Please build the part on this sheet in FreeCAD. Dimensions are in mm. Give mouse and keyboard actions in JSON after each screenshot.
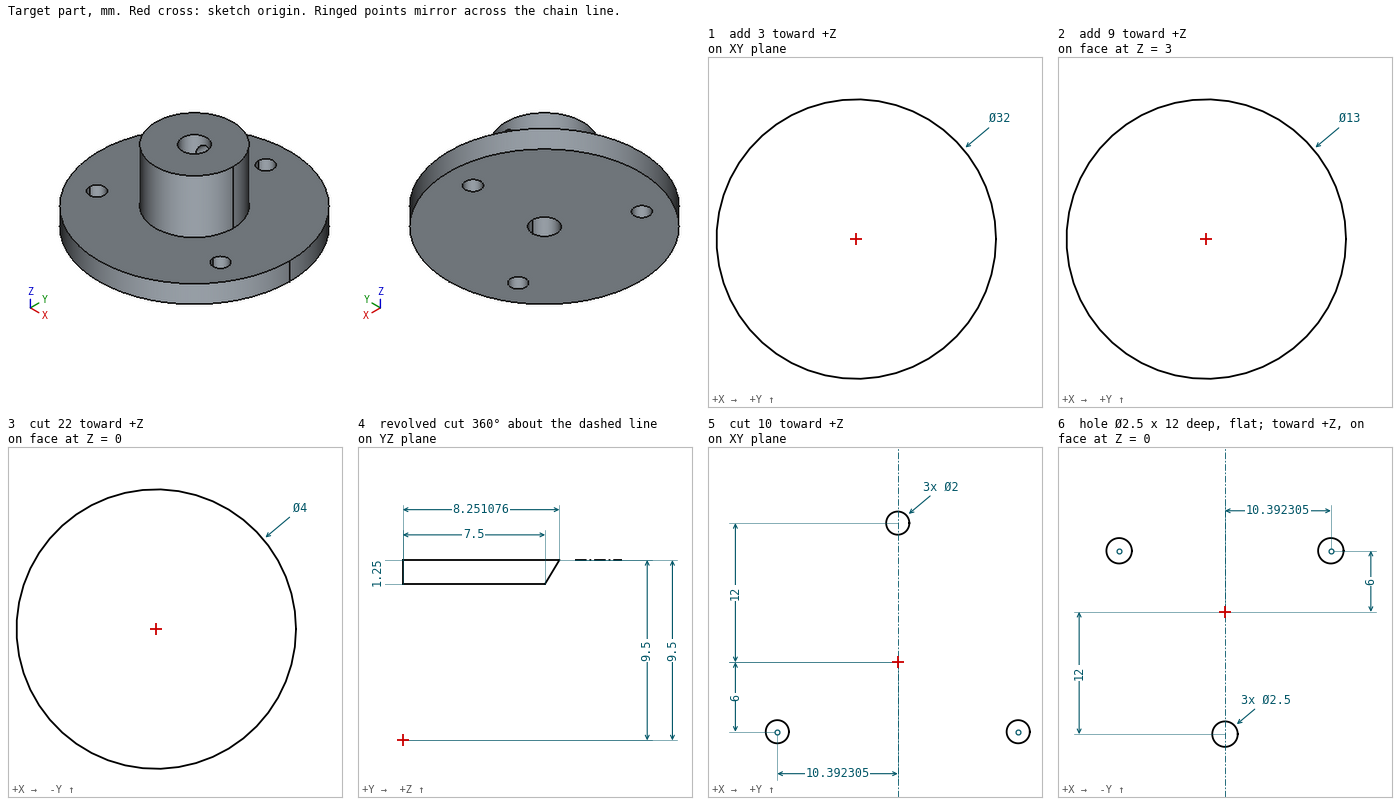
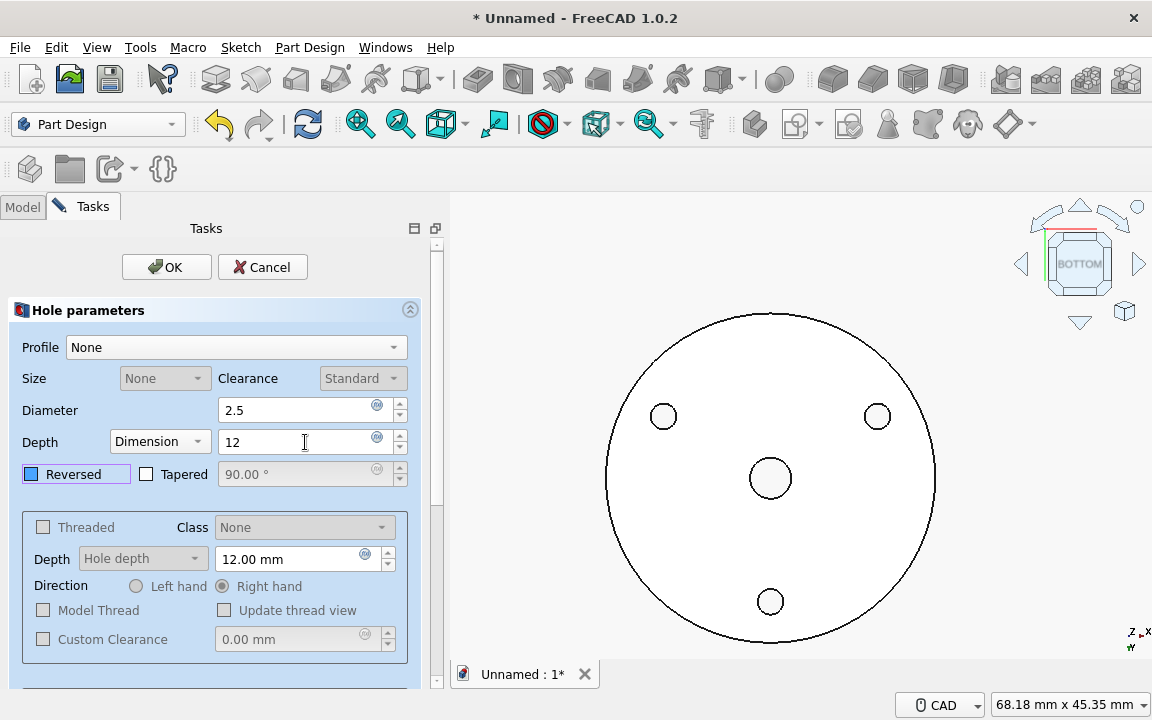
{"action": "scroll", "coordinate": [437, 463], "scroll_direction": "down", "scroll_amount": 5}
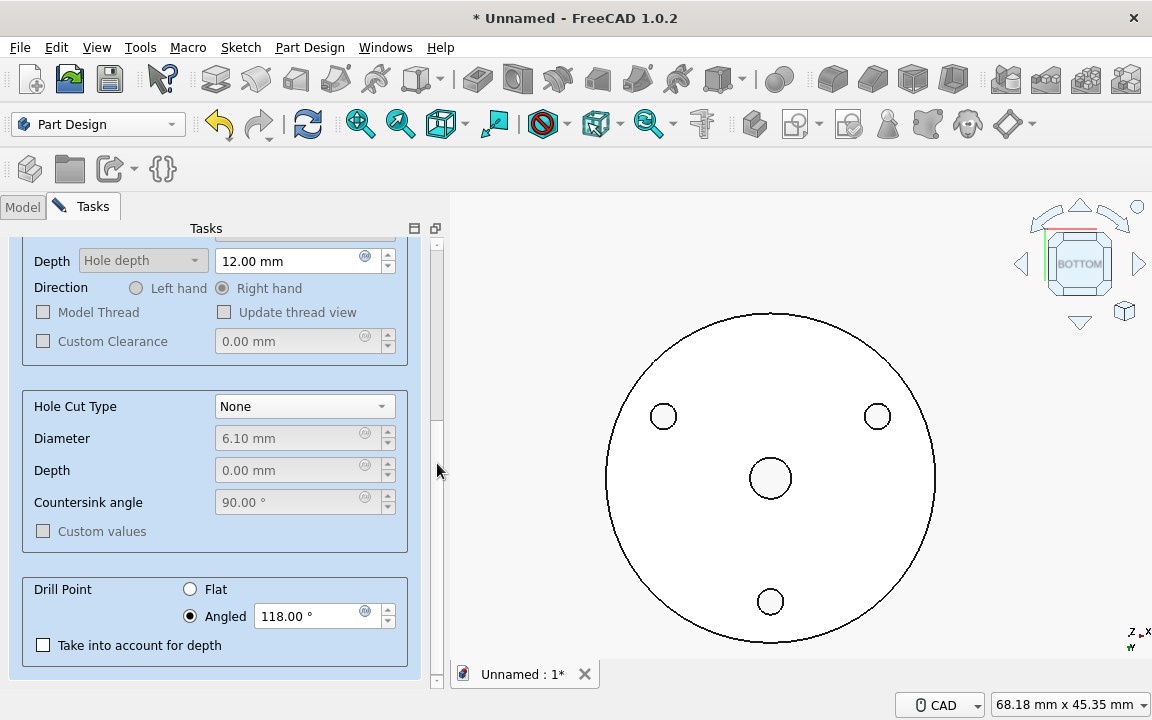
{"action": "left_click", "coordinate": [191, 589]}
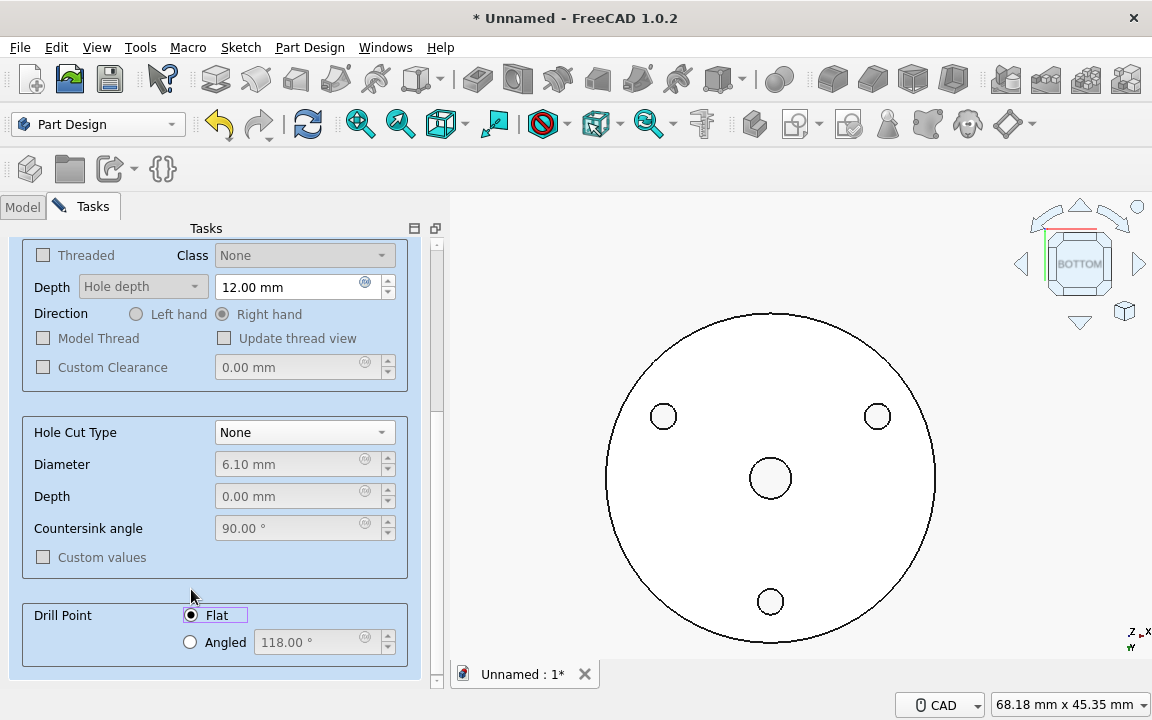
{"action": "scroll", "coordinate": [437, 463], "scroll_direction": "up", "scroll_amount": 6}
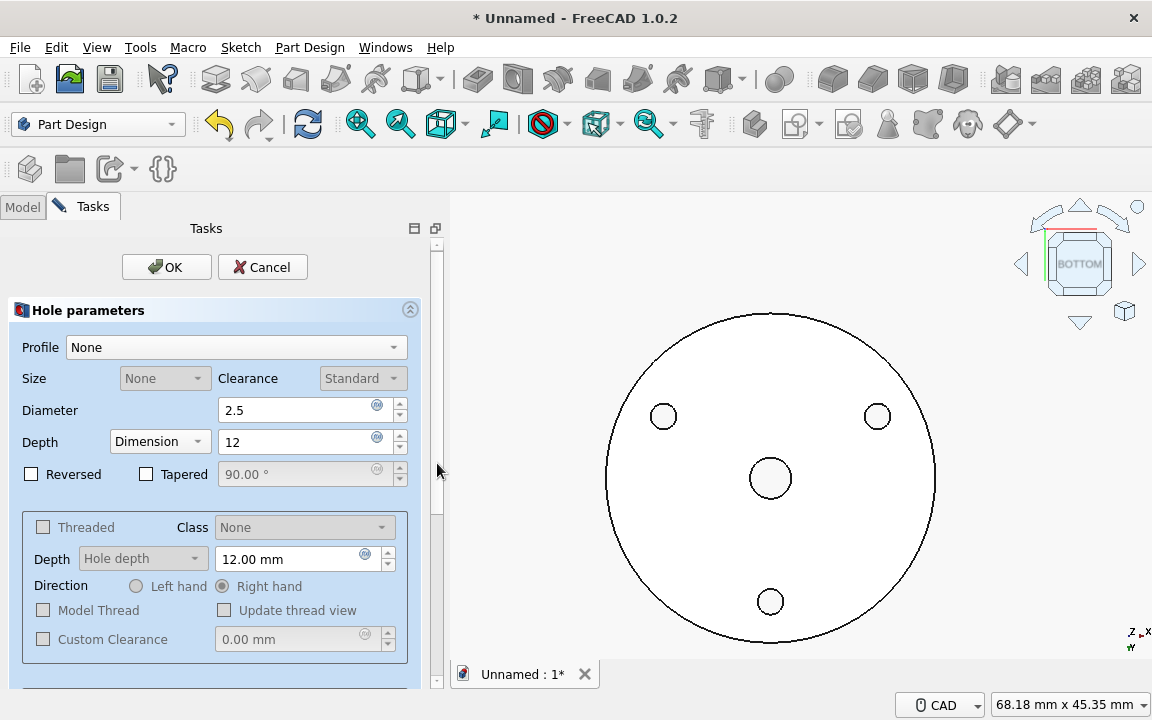
{"action": "left_click", "coordinate": [167, 267]}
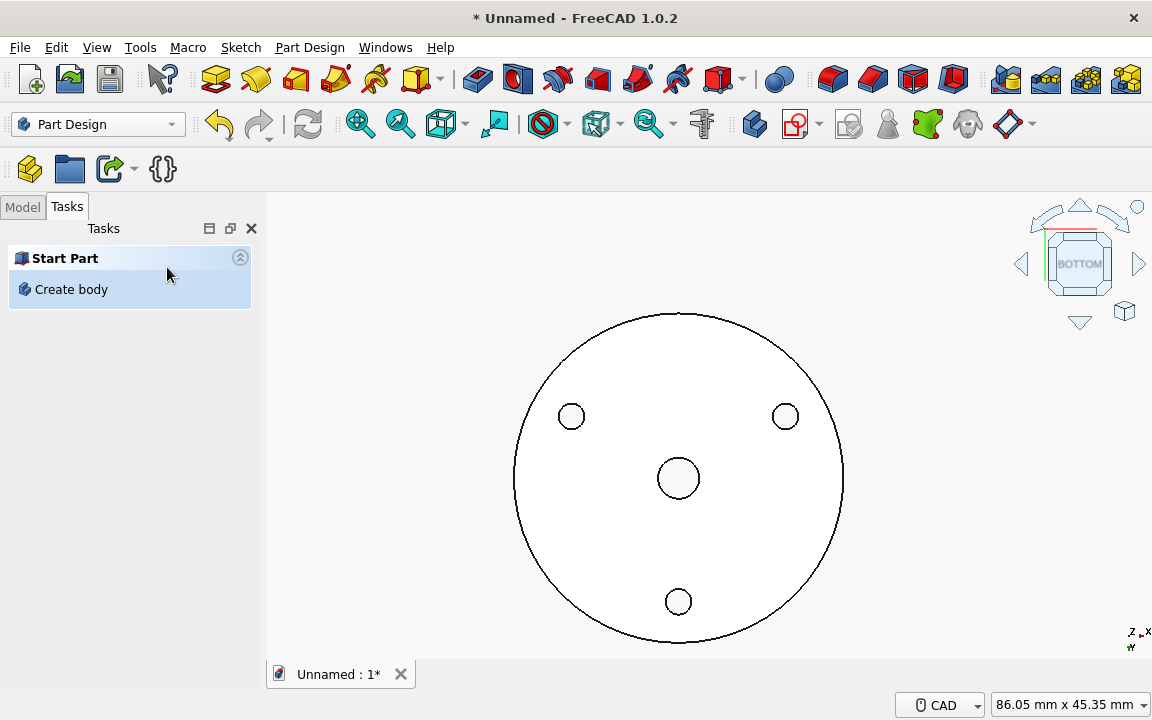
{"action": "key", "text": "0"}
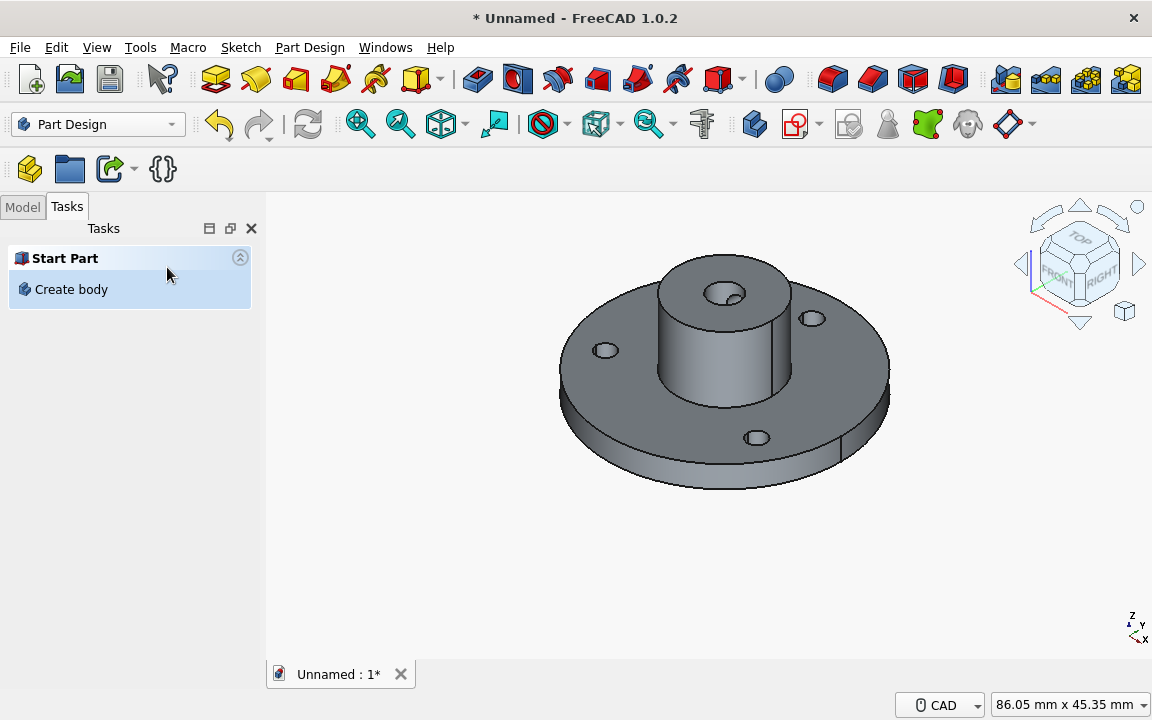
{"action": "left_click", "coordinate": [362, 124]}